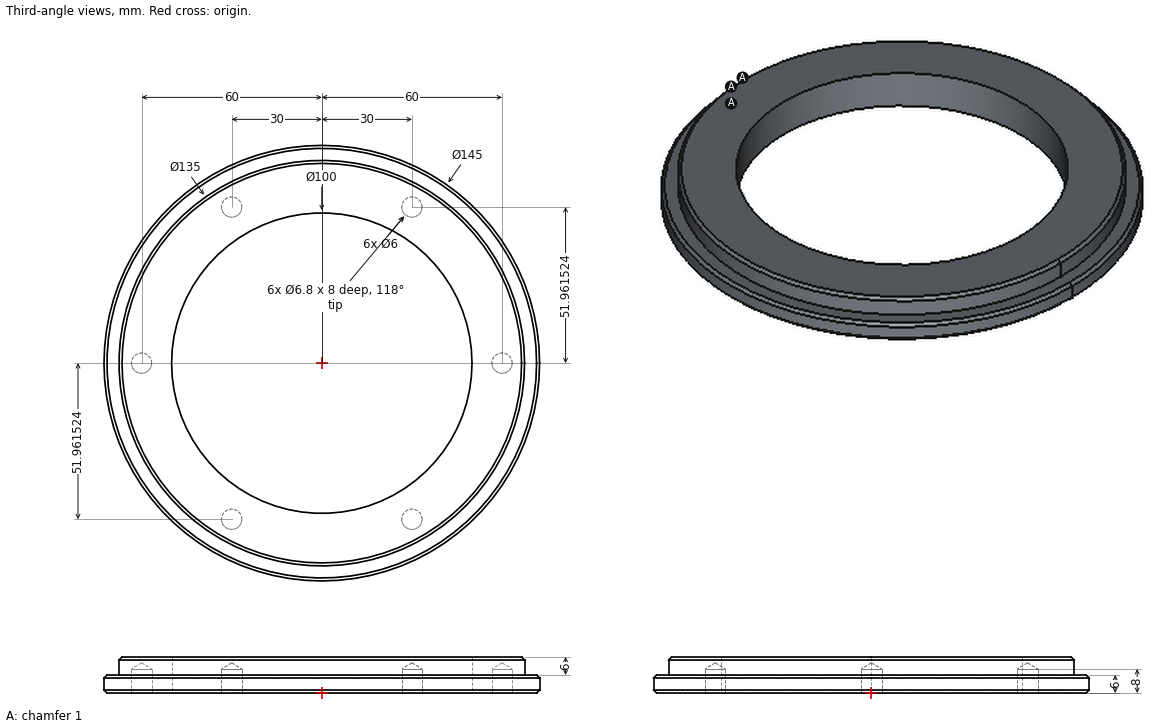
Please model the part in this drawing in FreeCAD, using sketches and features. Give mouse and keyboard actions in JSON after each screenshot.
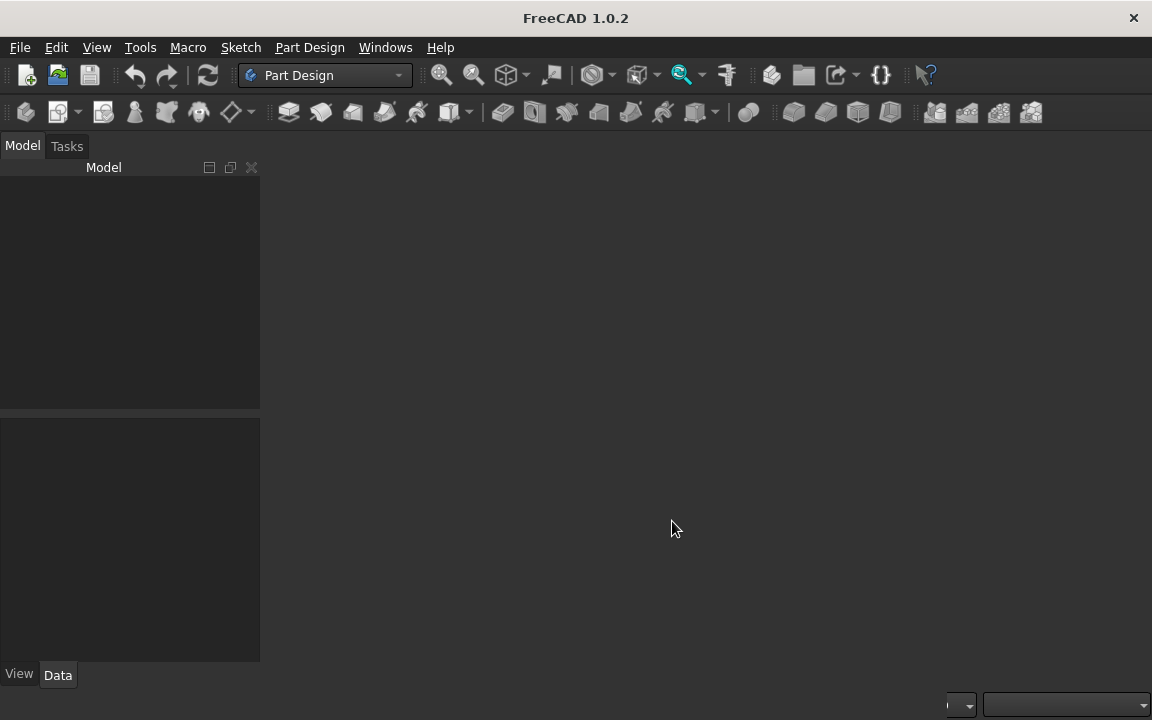
{"action": "left_click", "coordinate": [26, 76]}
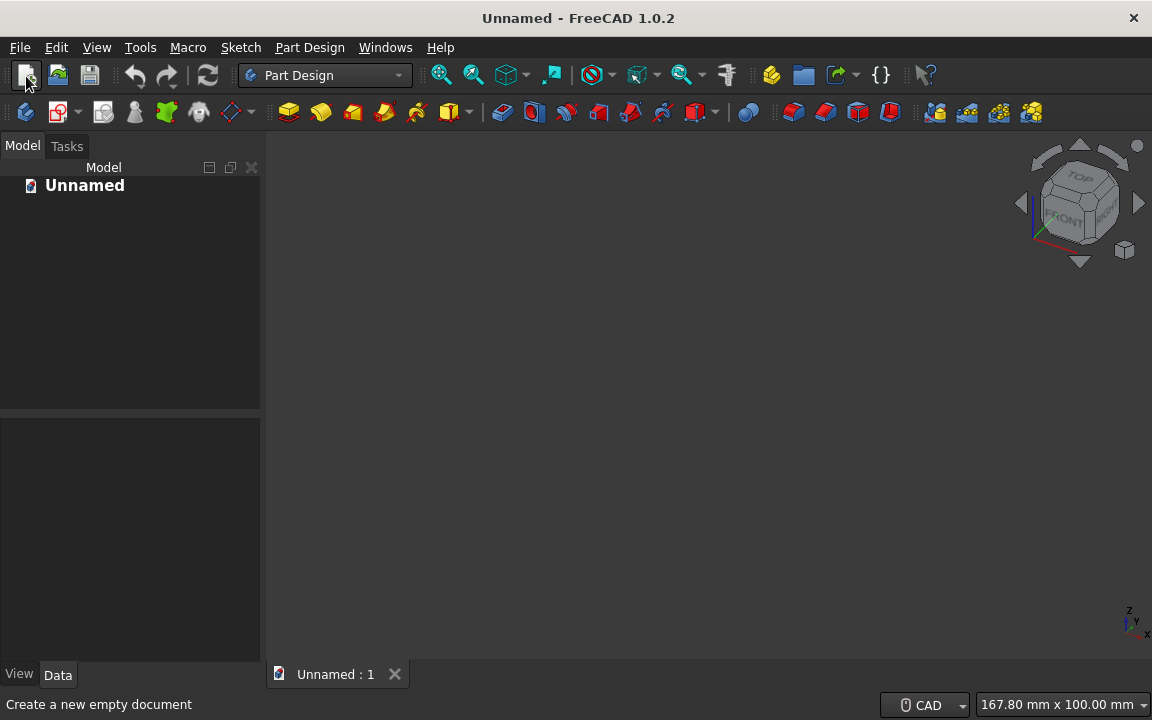
{"action": "left_click", "coordinate": [58, 112]}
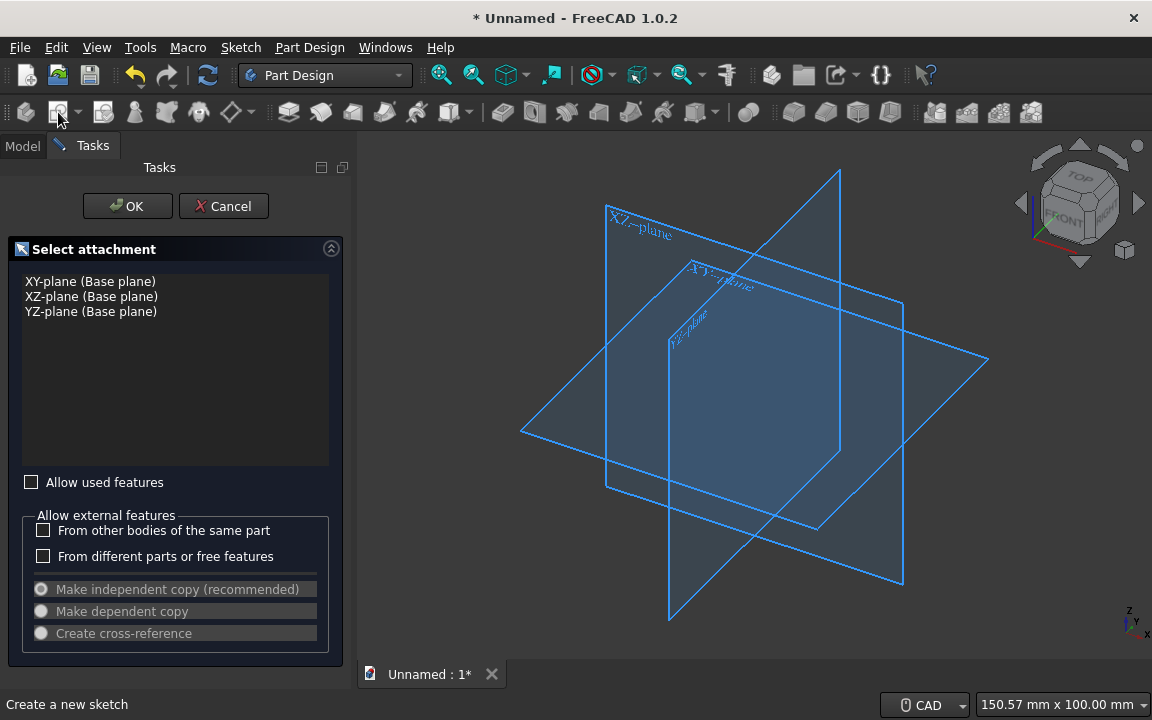
{"action": "left_click", "coordinate": [82, 282]}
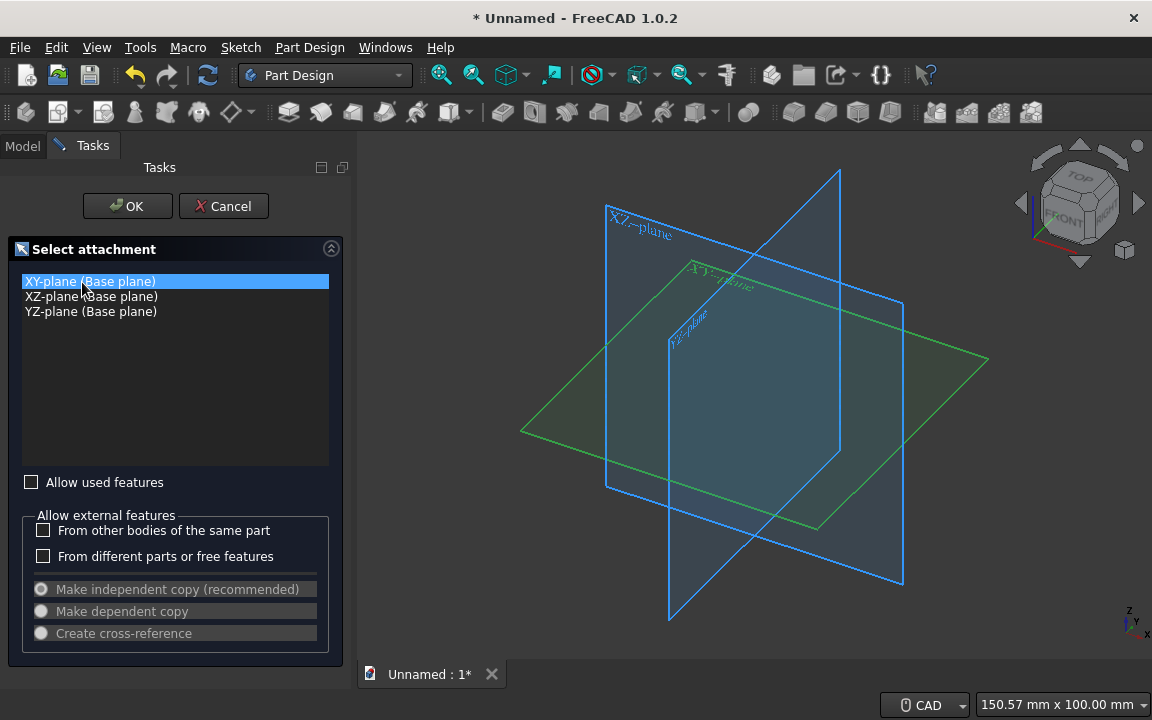
{"action": "left_click", "coordinate": [128, 206]}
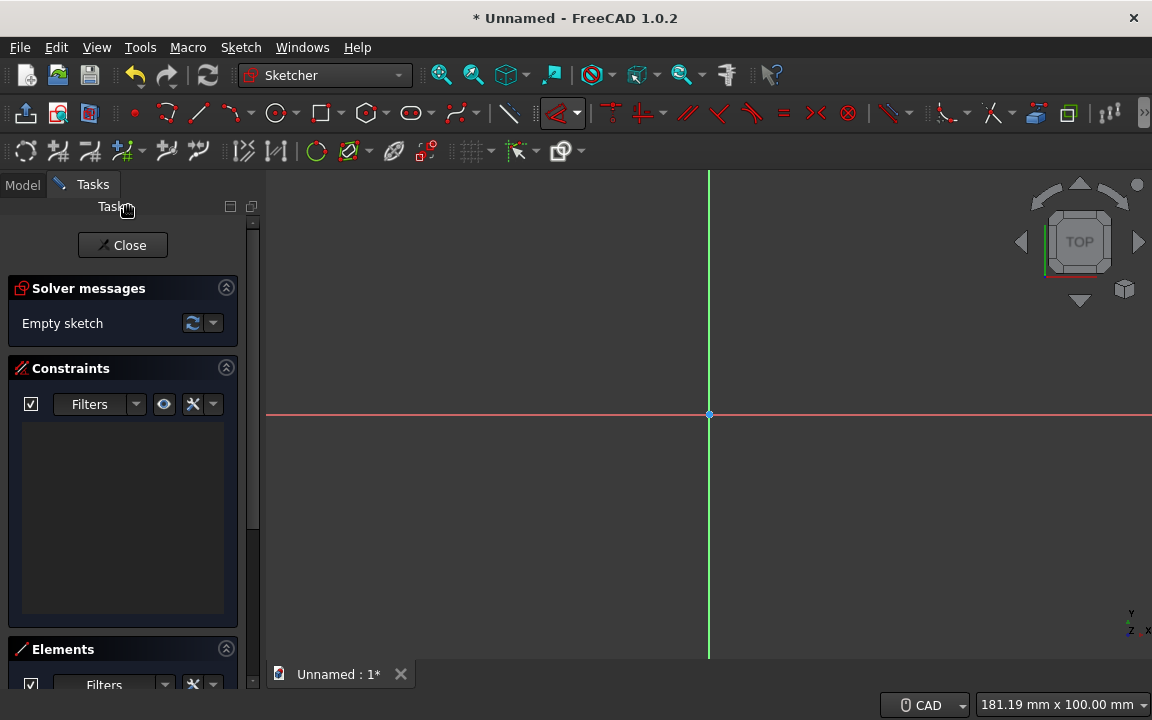
{"action": "scroll", "coordinate": [585, 414], "scroll_direction": "down", "scroll_amount": 4}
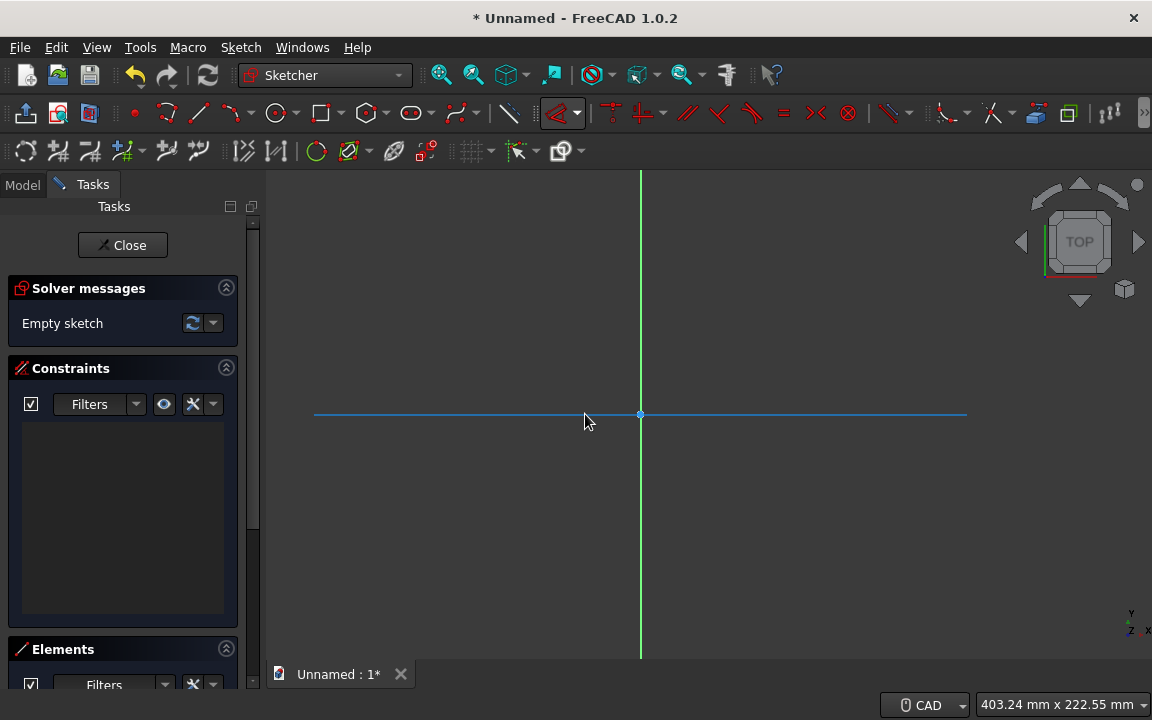
{"action": "left_click", "coordinate": [276, 114]}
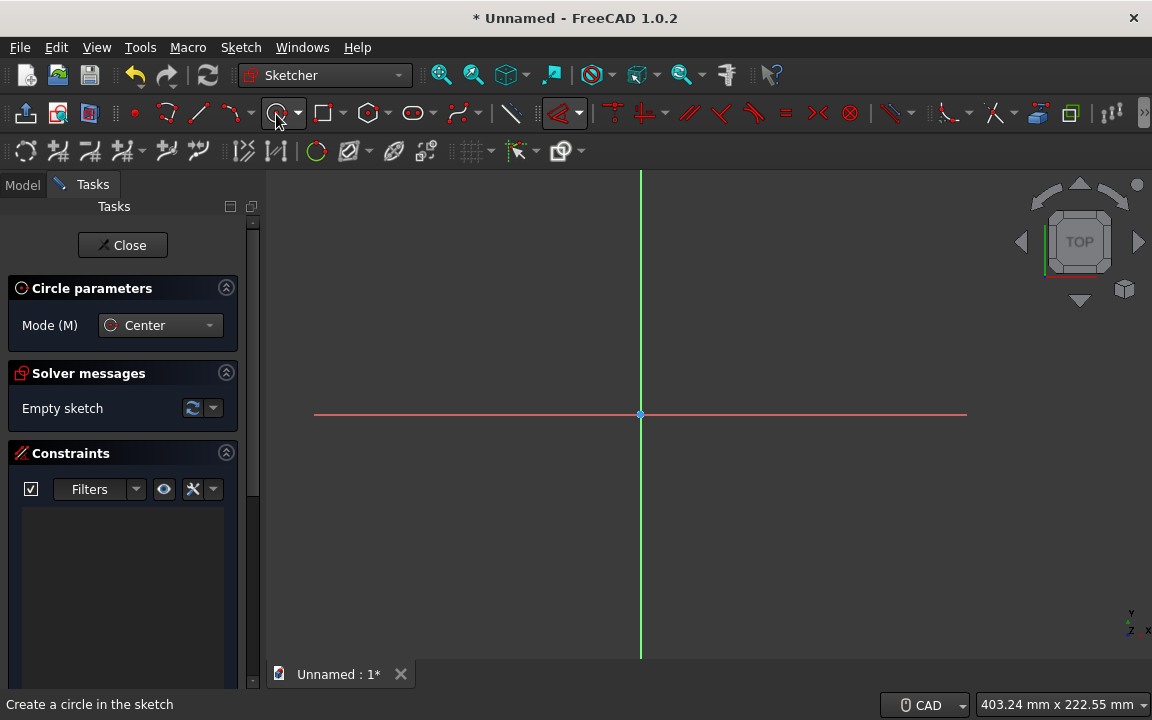
{"action": "left_click", "coordinate": [641, 414]}
{"action": "mouse_move", "coordinate": [754, 302]}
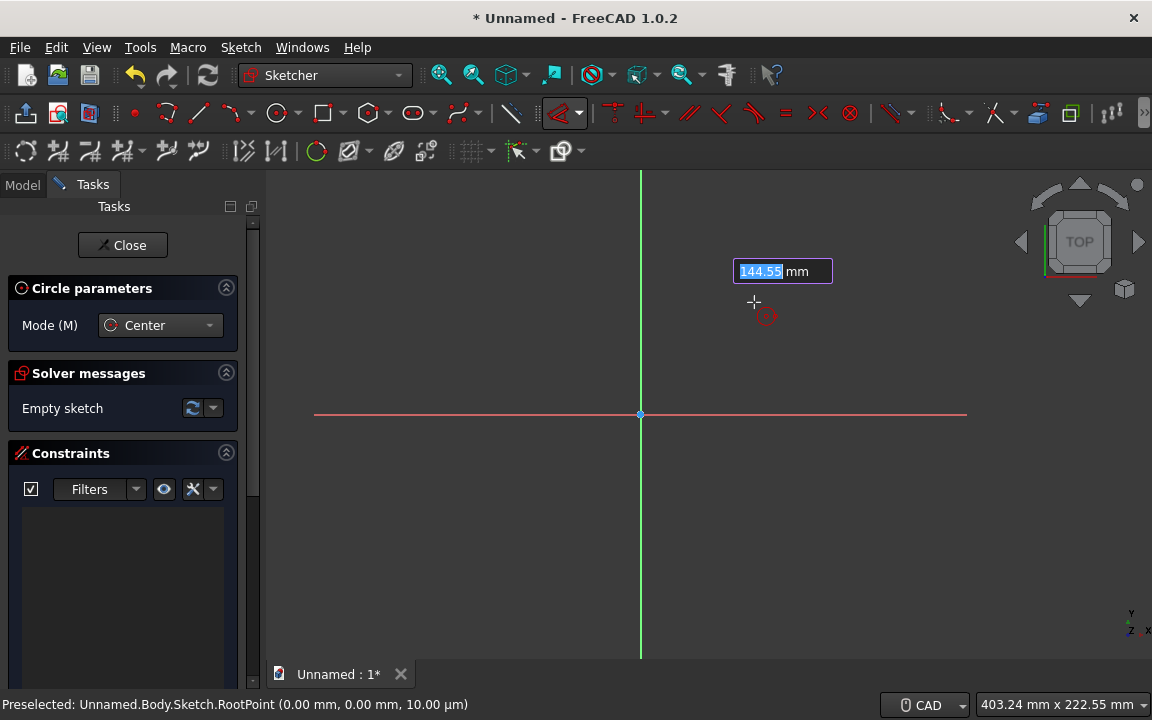
{"action": "type", "text": "145"}
{"action": "key", "text": "Return"}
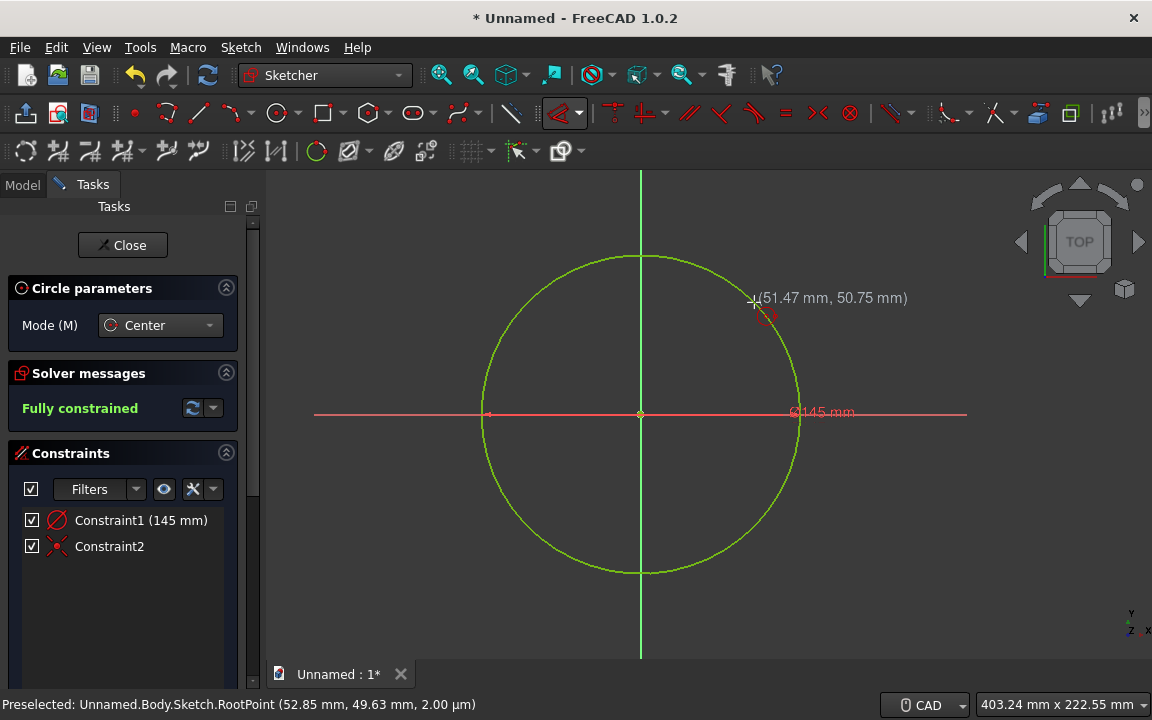
{"action": "left_click", "coordinate": [641, 414]}
{"action": "mouse_move", "coordinate": [719, 337]}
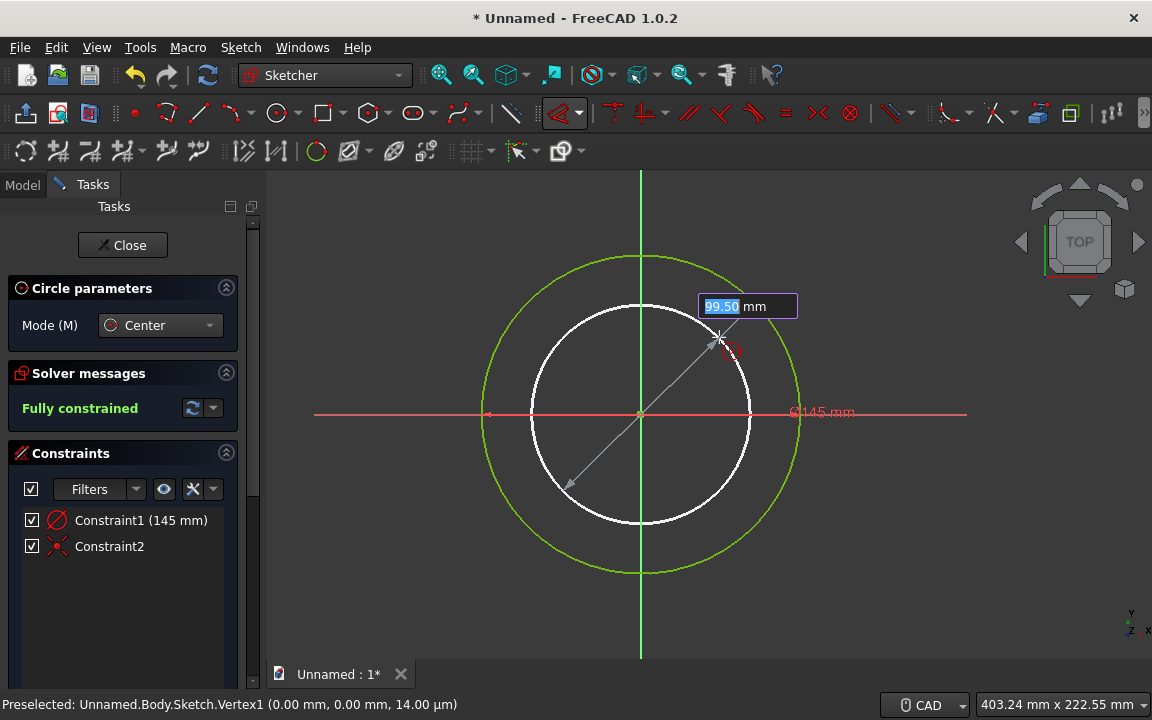
{"action": "type", "text": "100"}
{"action": "key", "text": "Return"}
{"action": "key", "text": "Escape"}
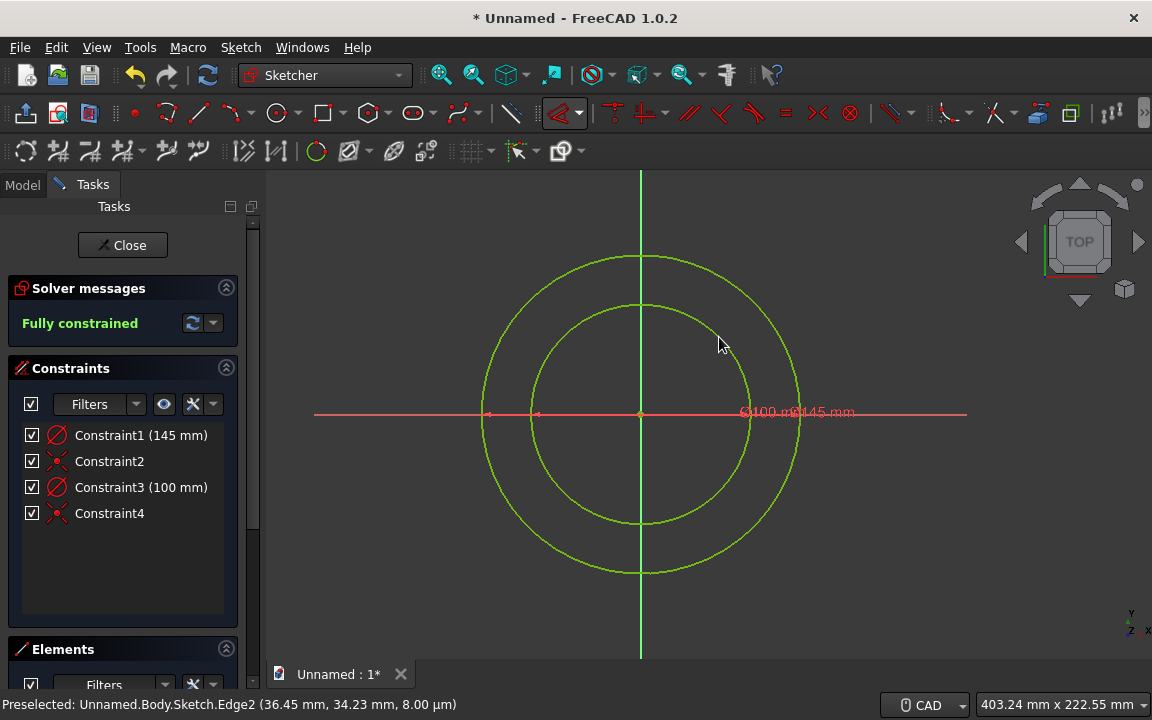
{"action": "left_click", "coordinate": [123, 245]}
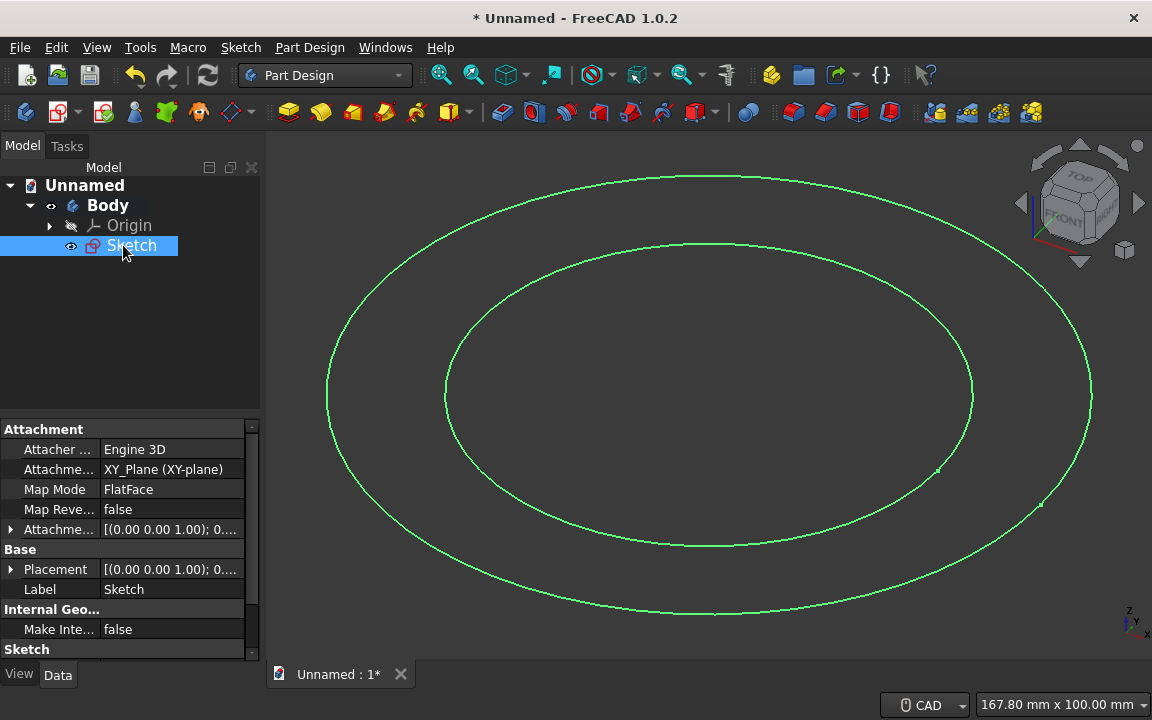
{"action": "left_click", "coordinate": [290, 112]}